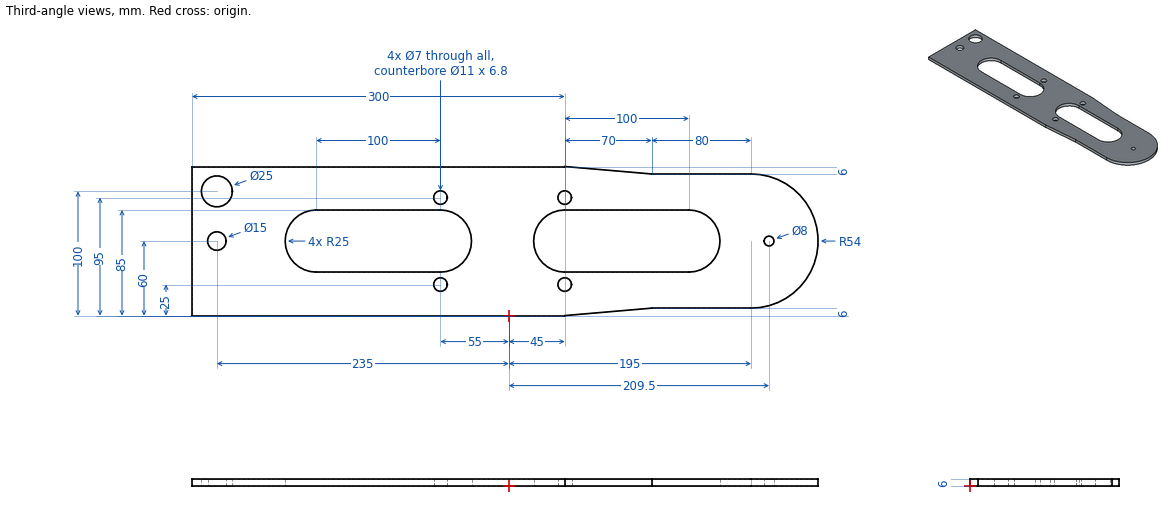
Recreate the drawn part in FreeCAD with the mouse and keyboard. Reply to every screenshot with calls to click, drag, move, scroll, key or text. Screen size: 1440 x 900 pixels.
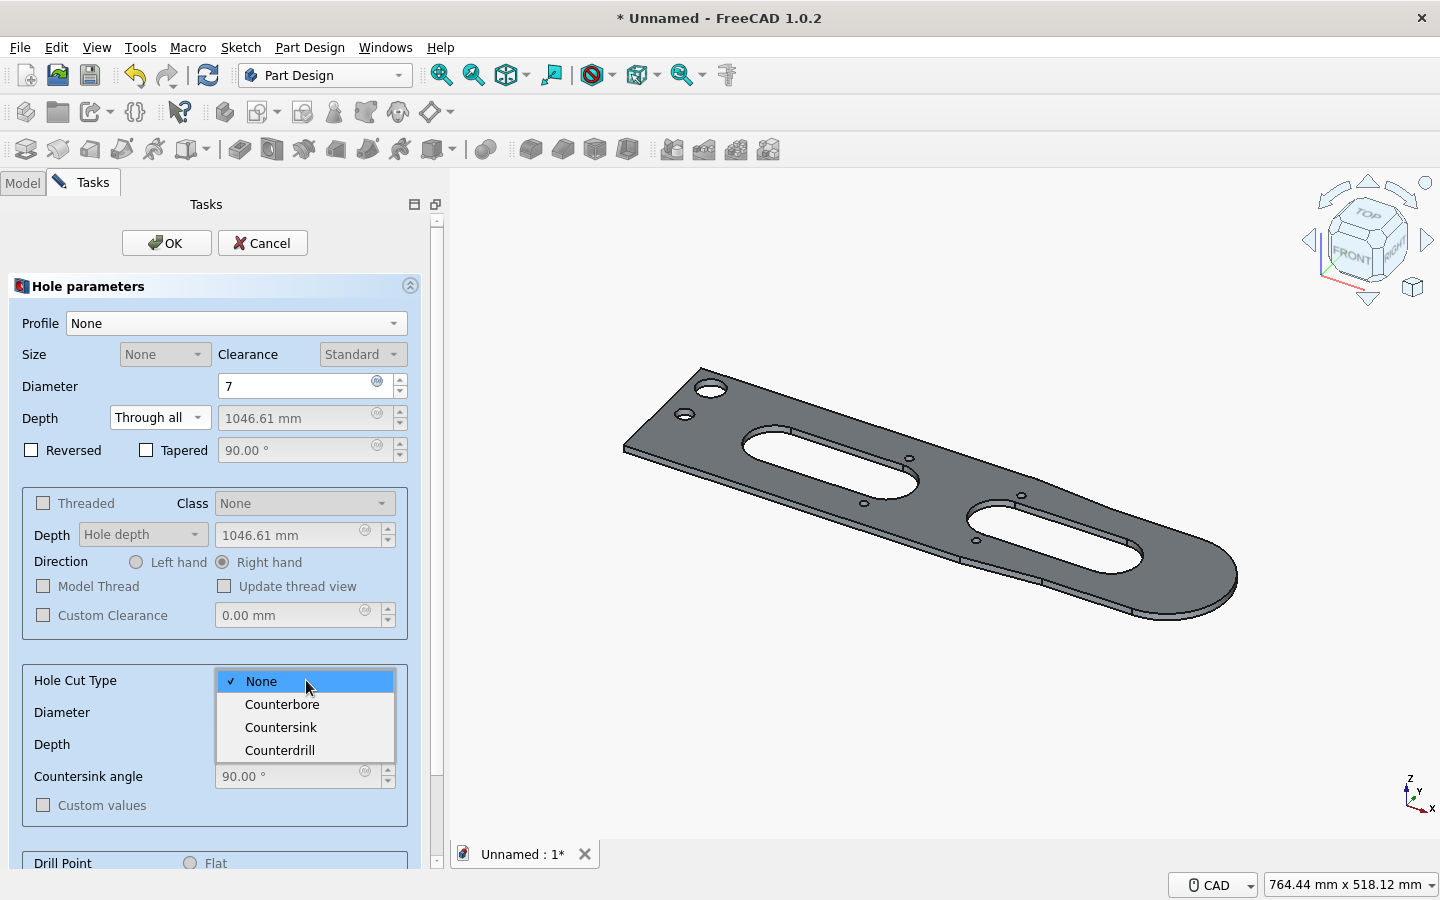
click(304, 704)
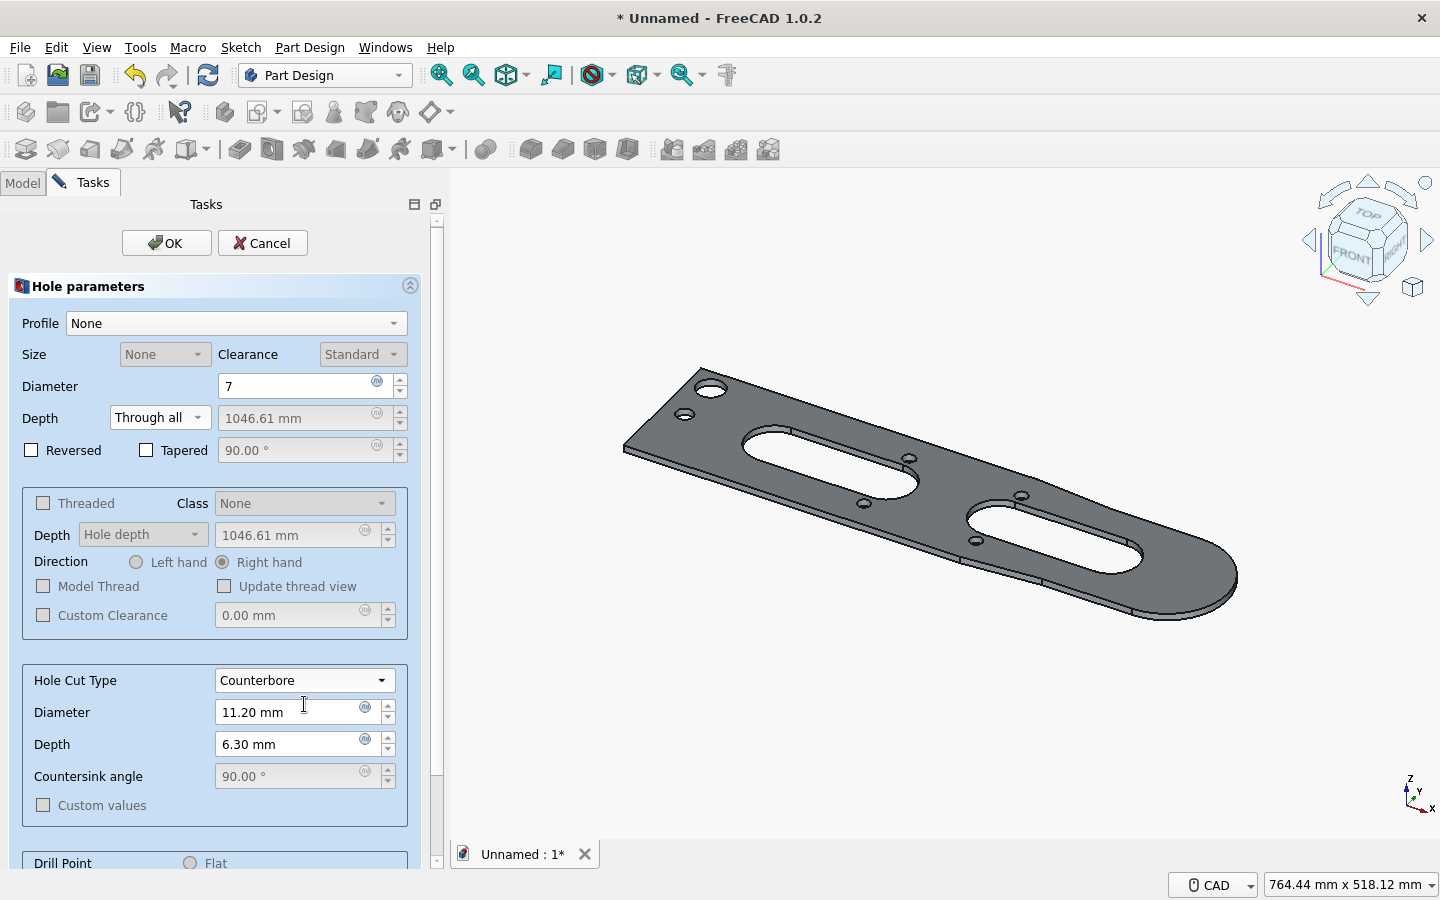
triple_click(298, 712)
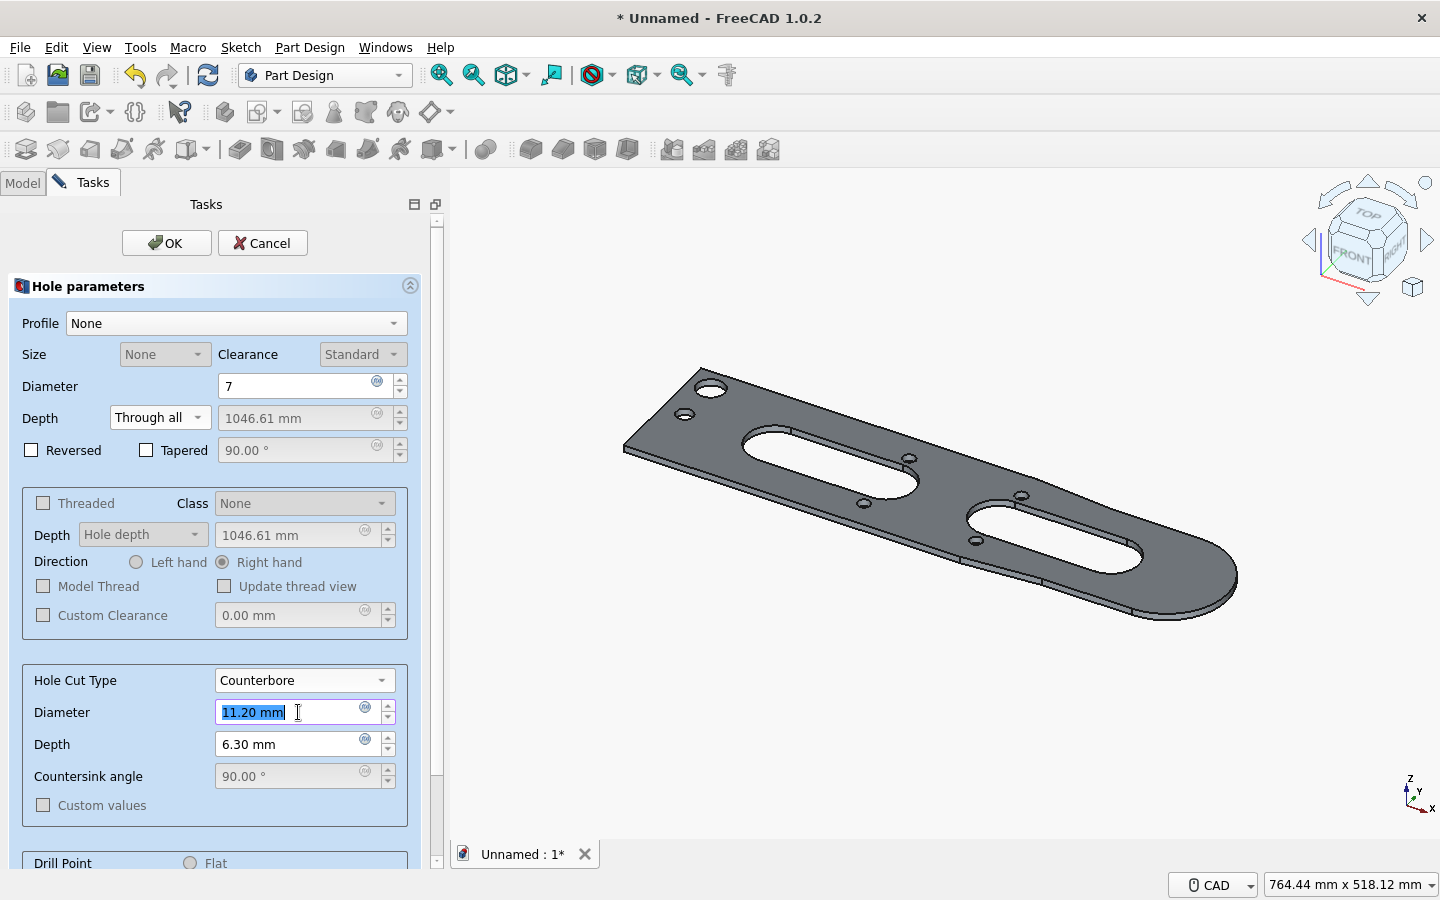
text(11)
key(Tab)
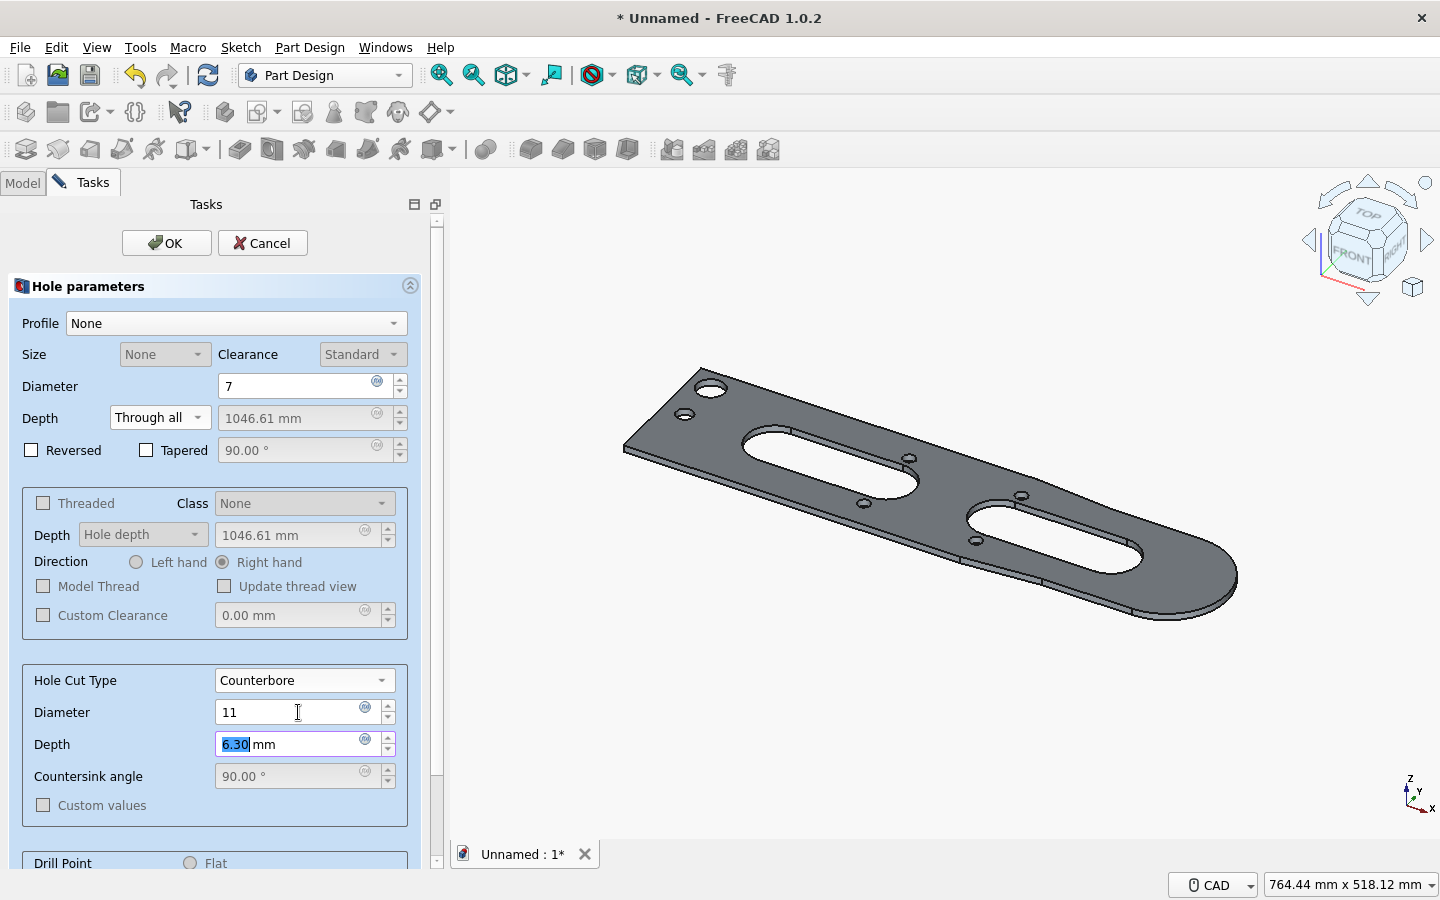
text(6.8)
key(Tab)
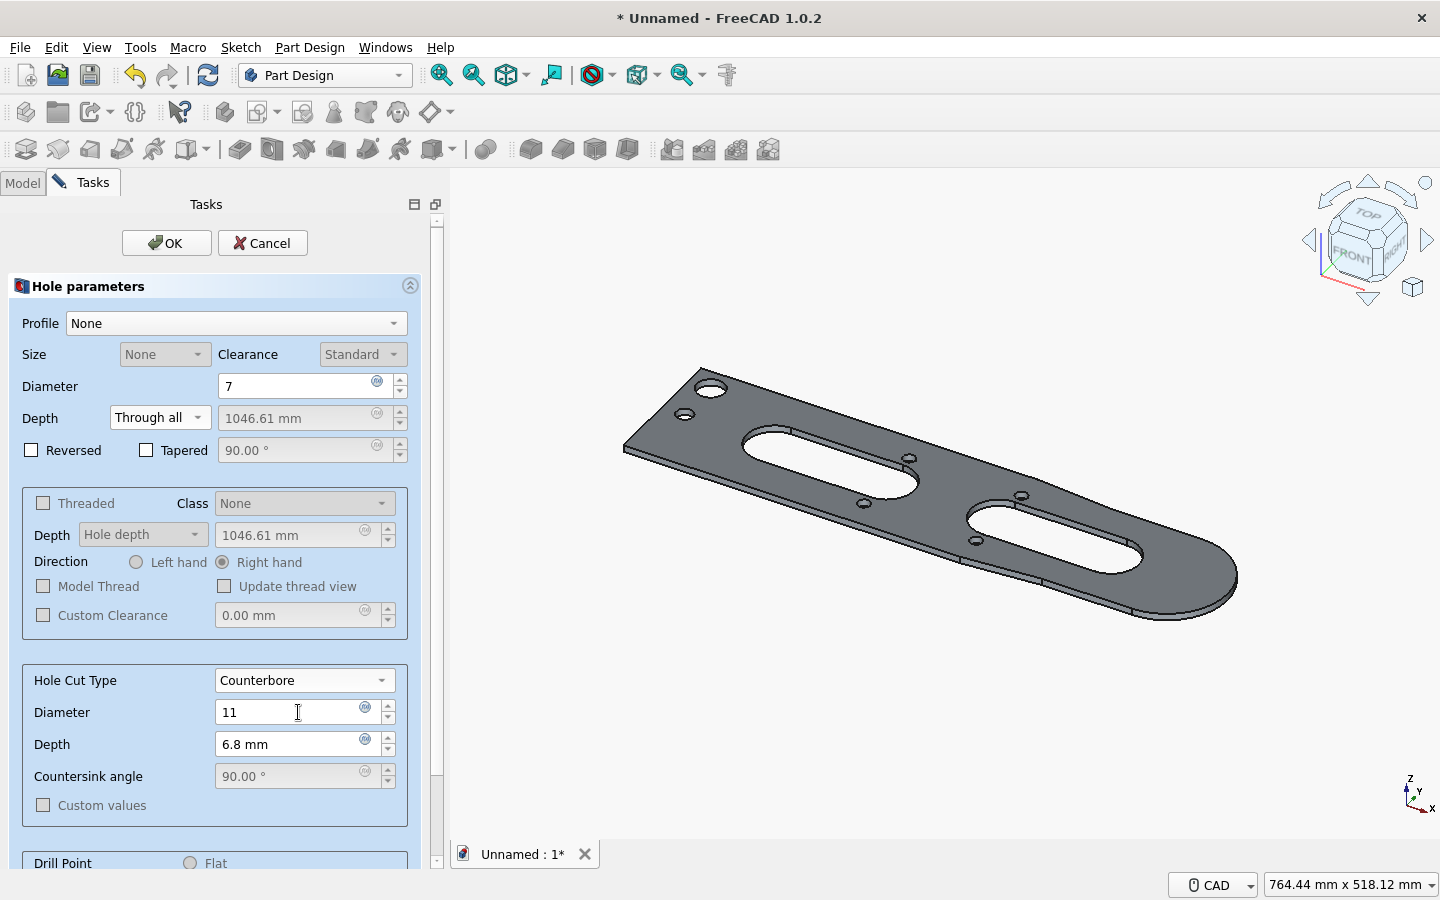
click(167, 243)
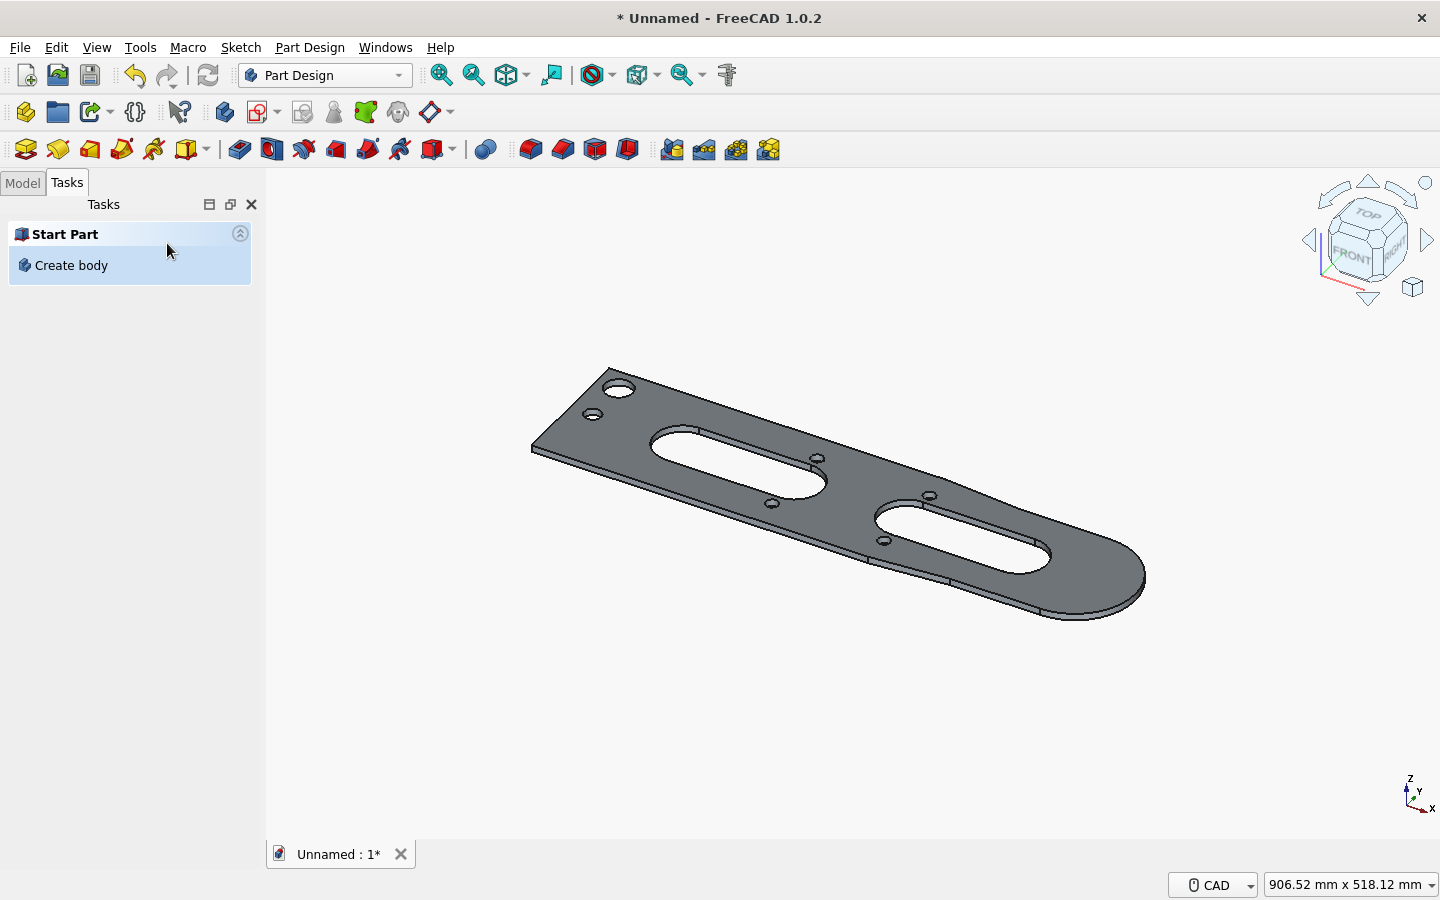
click(258, 112)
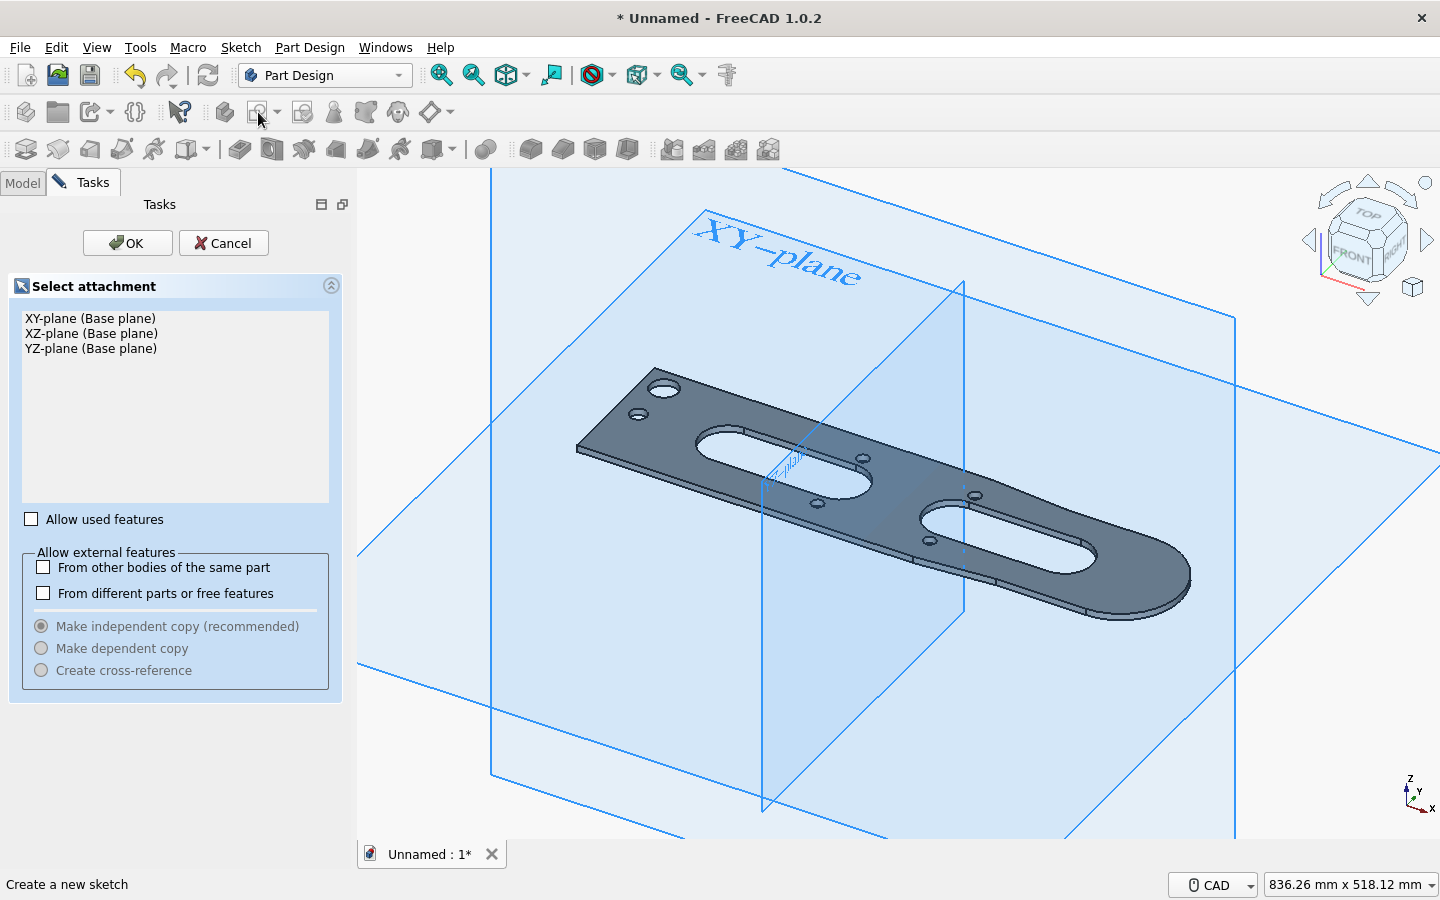
click(82, 318)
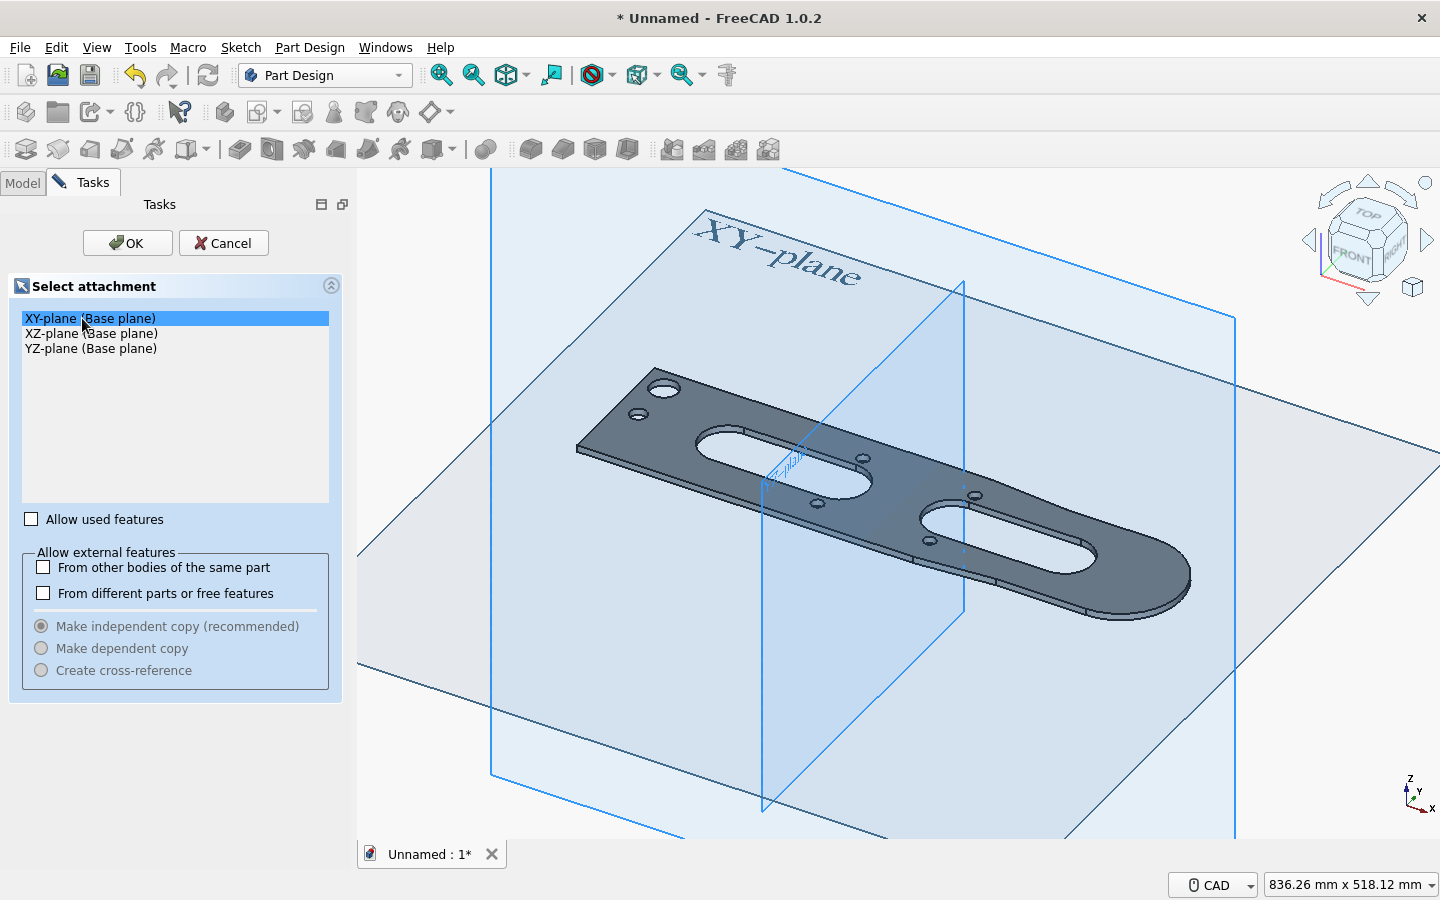
click(128, 243)